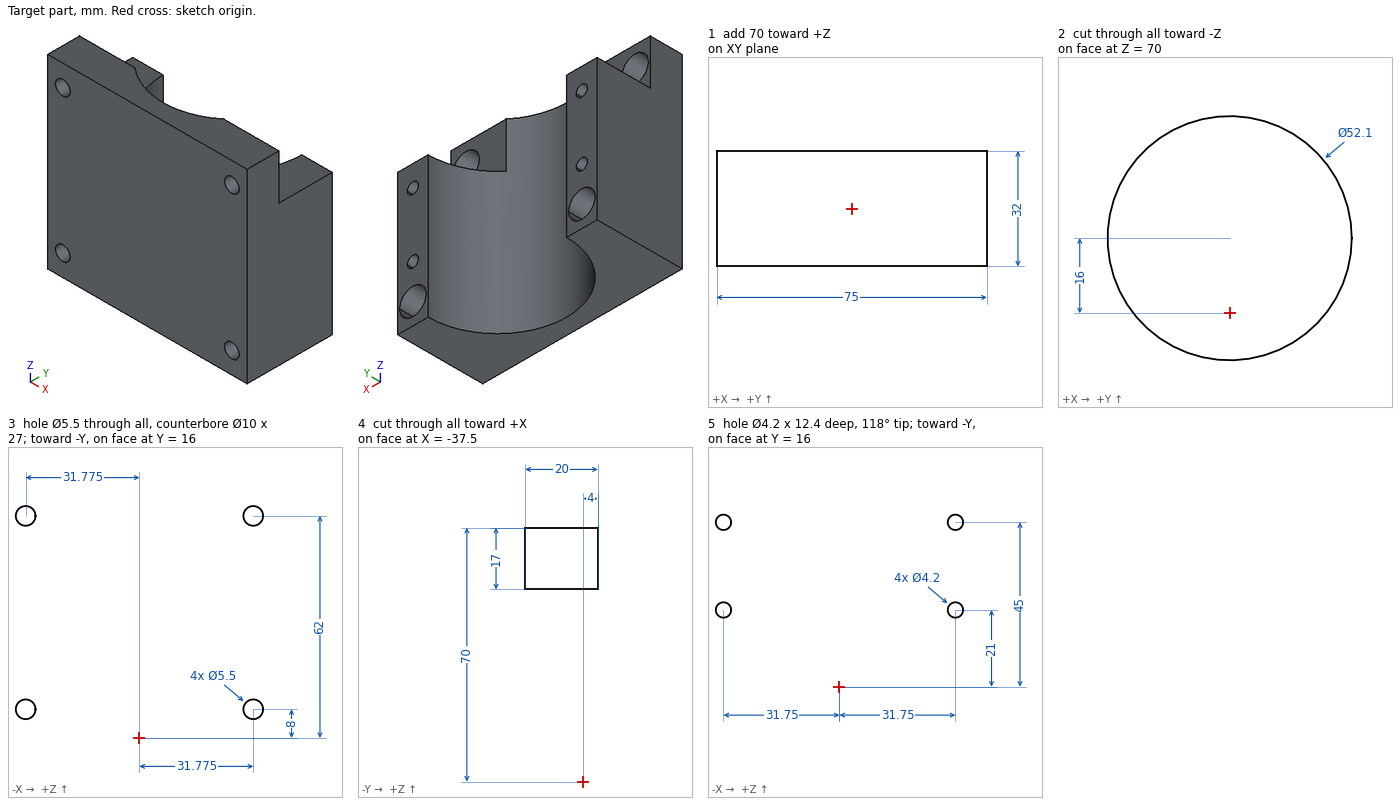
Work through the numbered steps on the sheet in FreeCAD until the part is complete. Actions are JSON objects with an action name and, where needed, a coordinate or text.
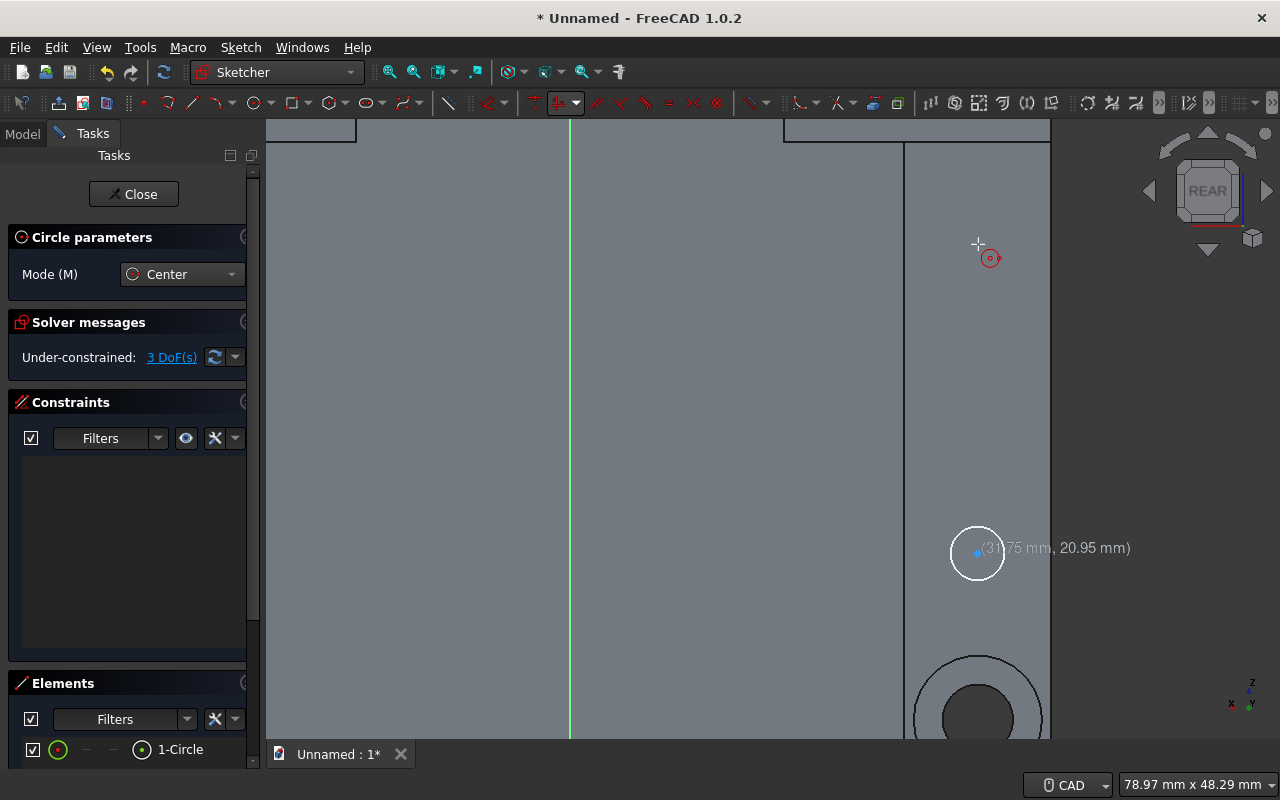
{"action": "left_click", "coordinate": [978, 245]}
{"action": "left_click", "coordinate": [997, 226]}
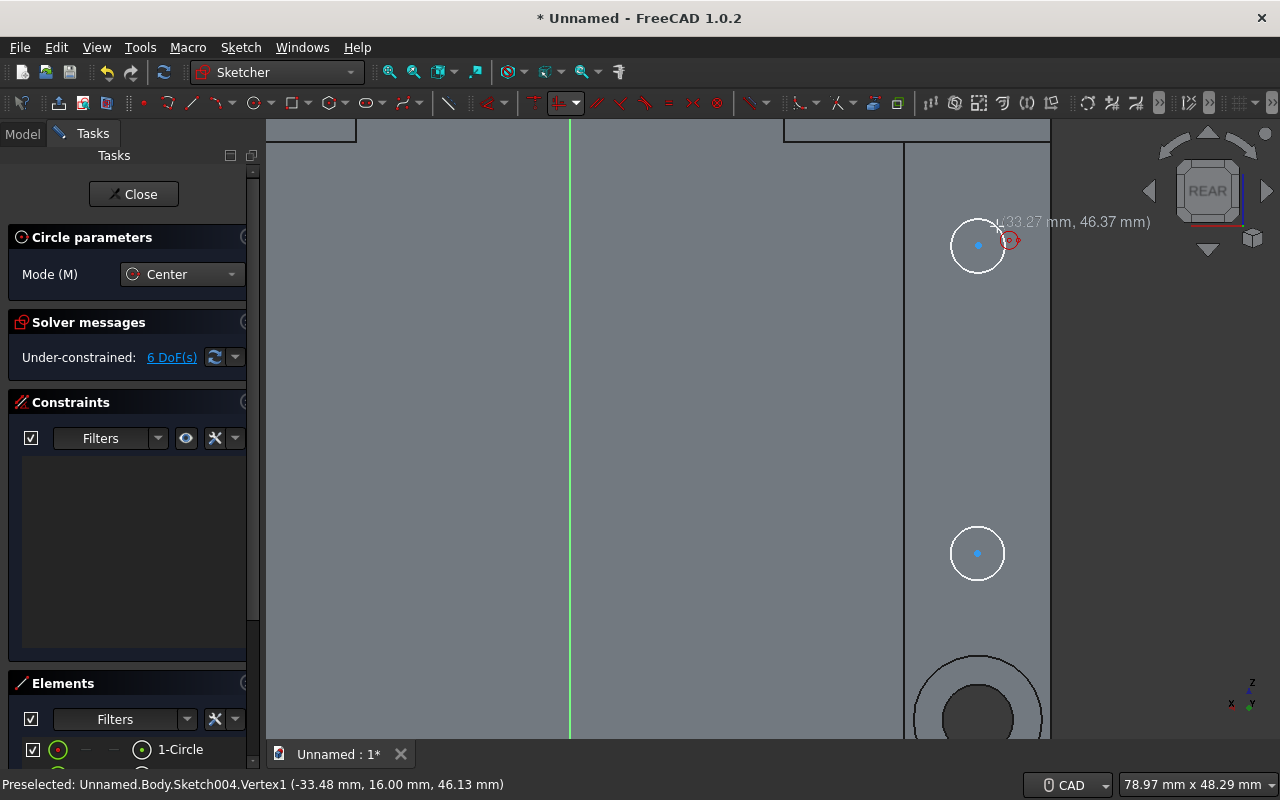
{"action": "scroll", "coordinate": [978, 244], "scroll_direction": "down", "scroll_amount": 2}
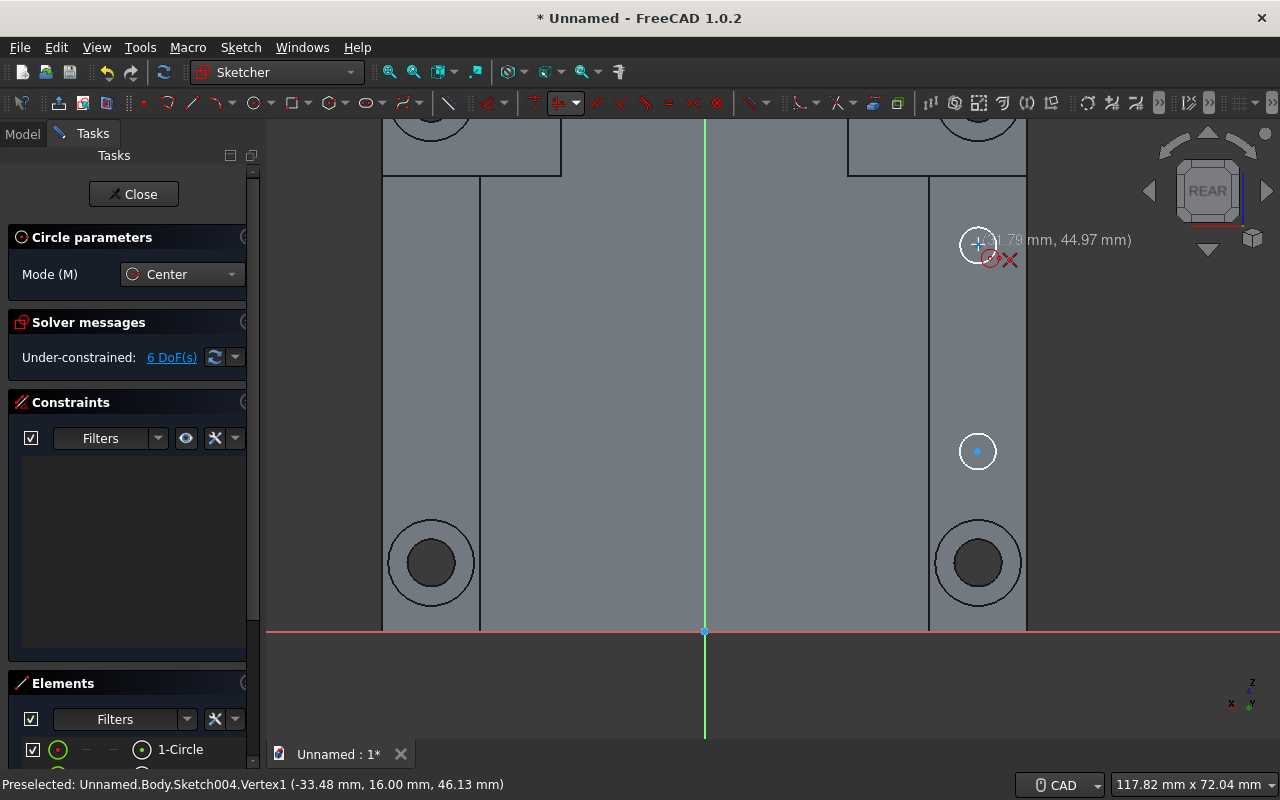
{"action": "scroll", "coordinate": [431, 451], "scroll_direction": "up", "scroll_amount": 2}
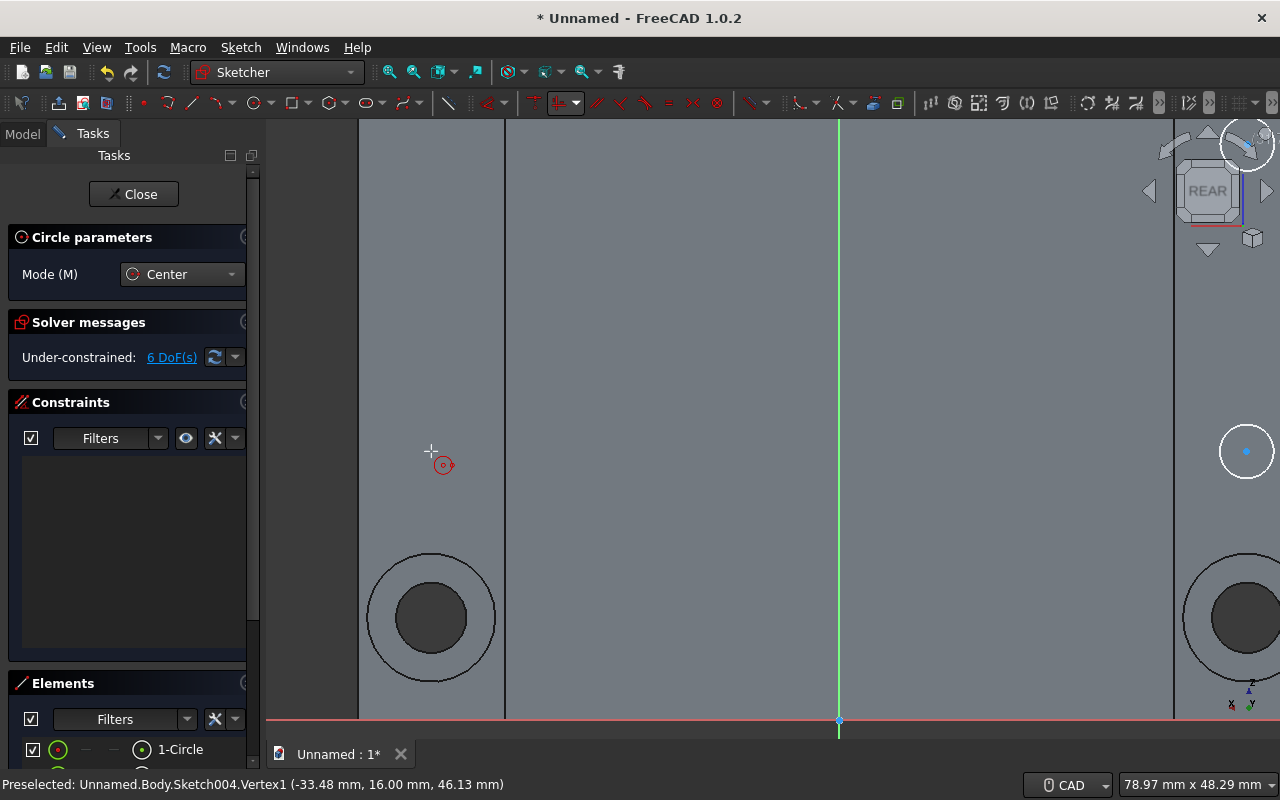
{"action": "left_click", "coordinate": [432, 451]}
{"action": "left_click", "coordinate": [451, 432]}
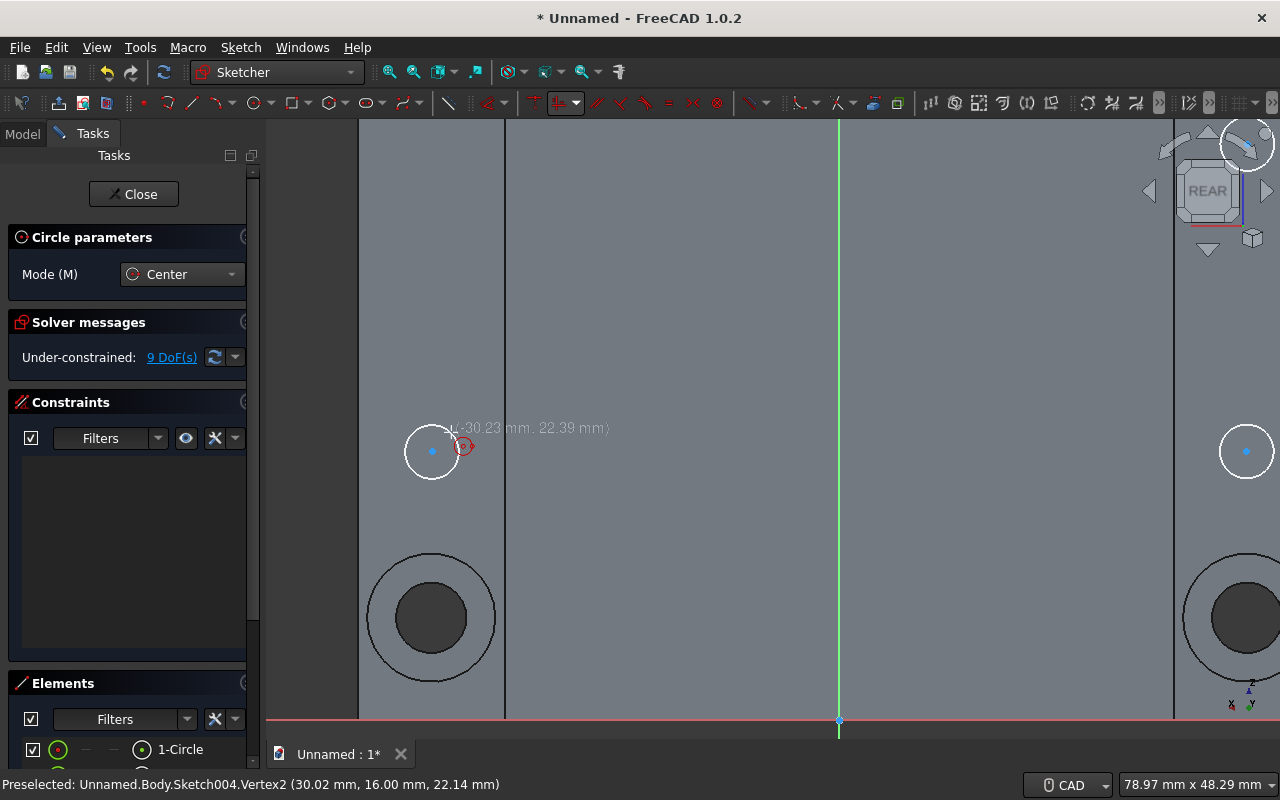
{"action": "scroll", "coordinate": [431, 451], "scroll_direction": "down", "scroll_amount": 2}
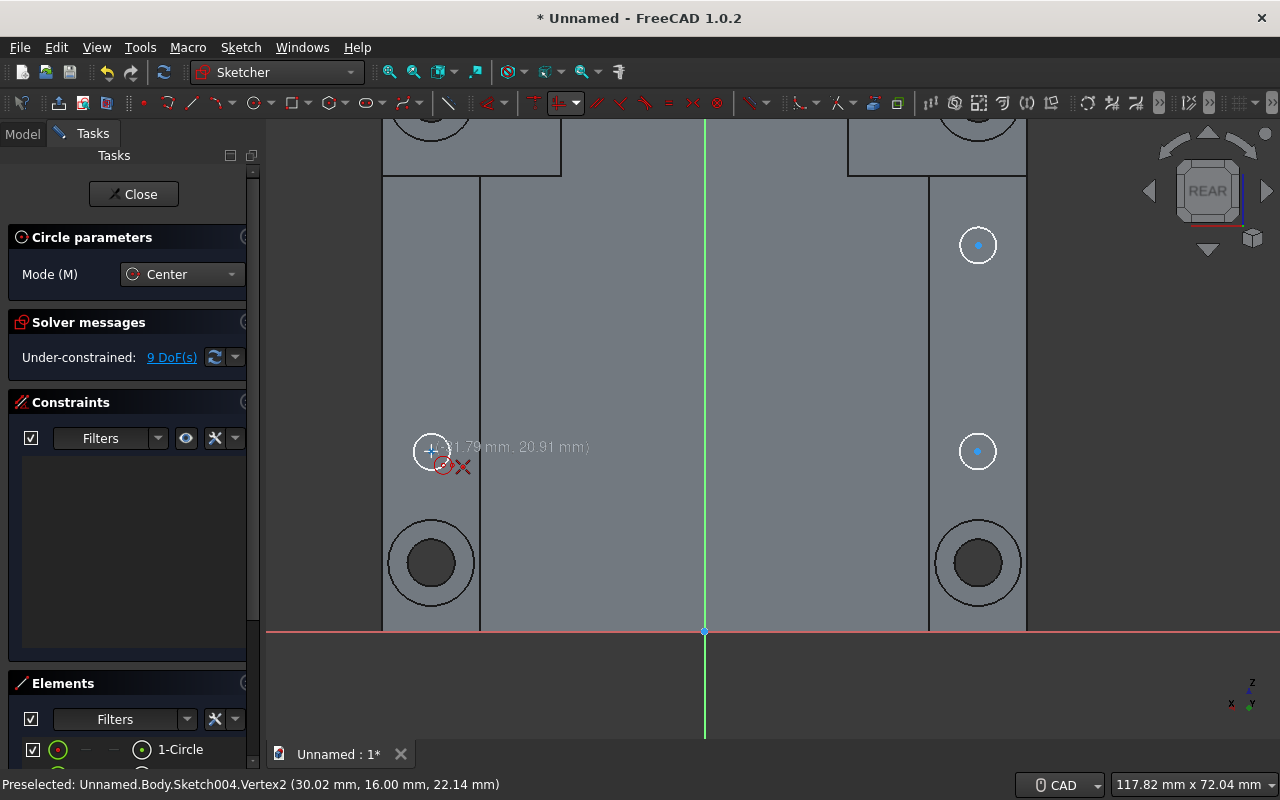
{"action": "scroll", "coordinate": [431, 244], "scroll_direction": "up", "scroll_amount": 2}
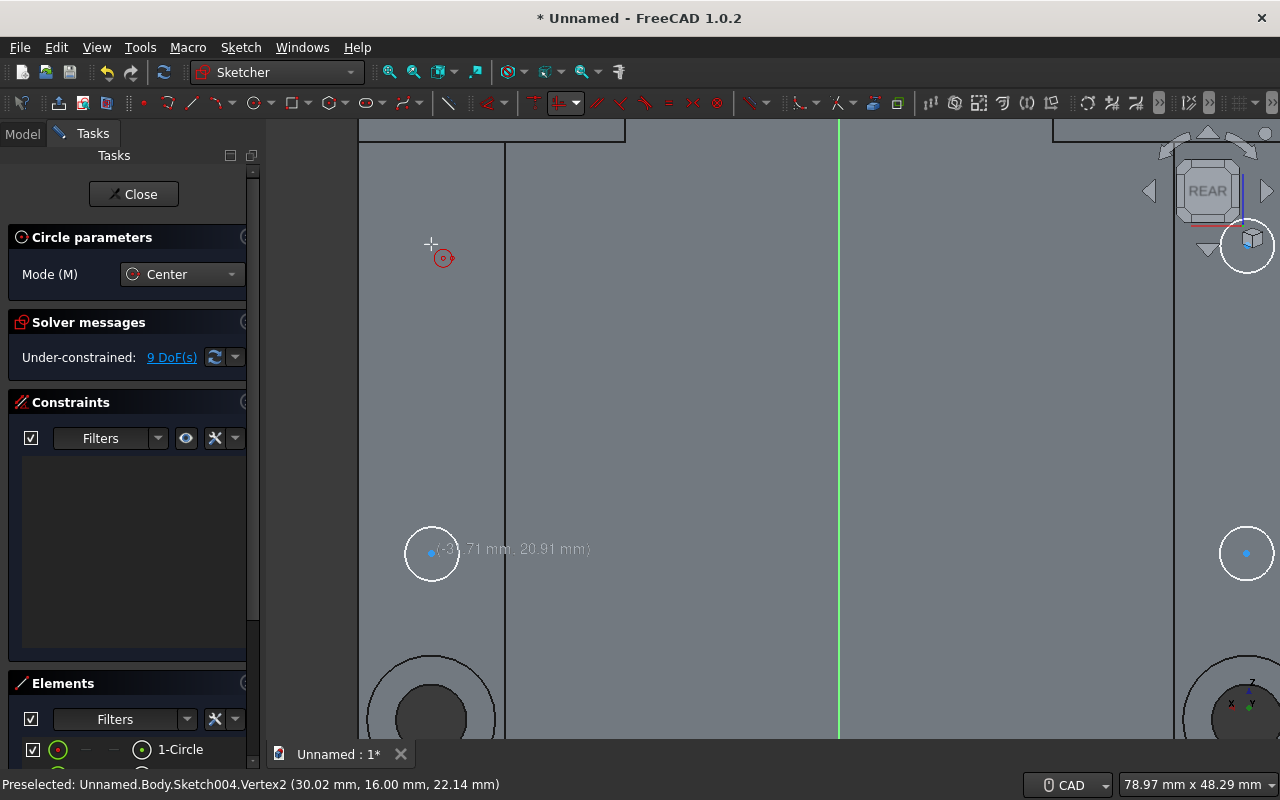
{"action": "left_click", "coordinate": [432, 245]}
{"action": "left_click", "coordinate": [451, 226]}
{"action": "key", "text": "Escape"}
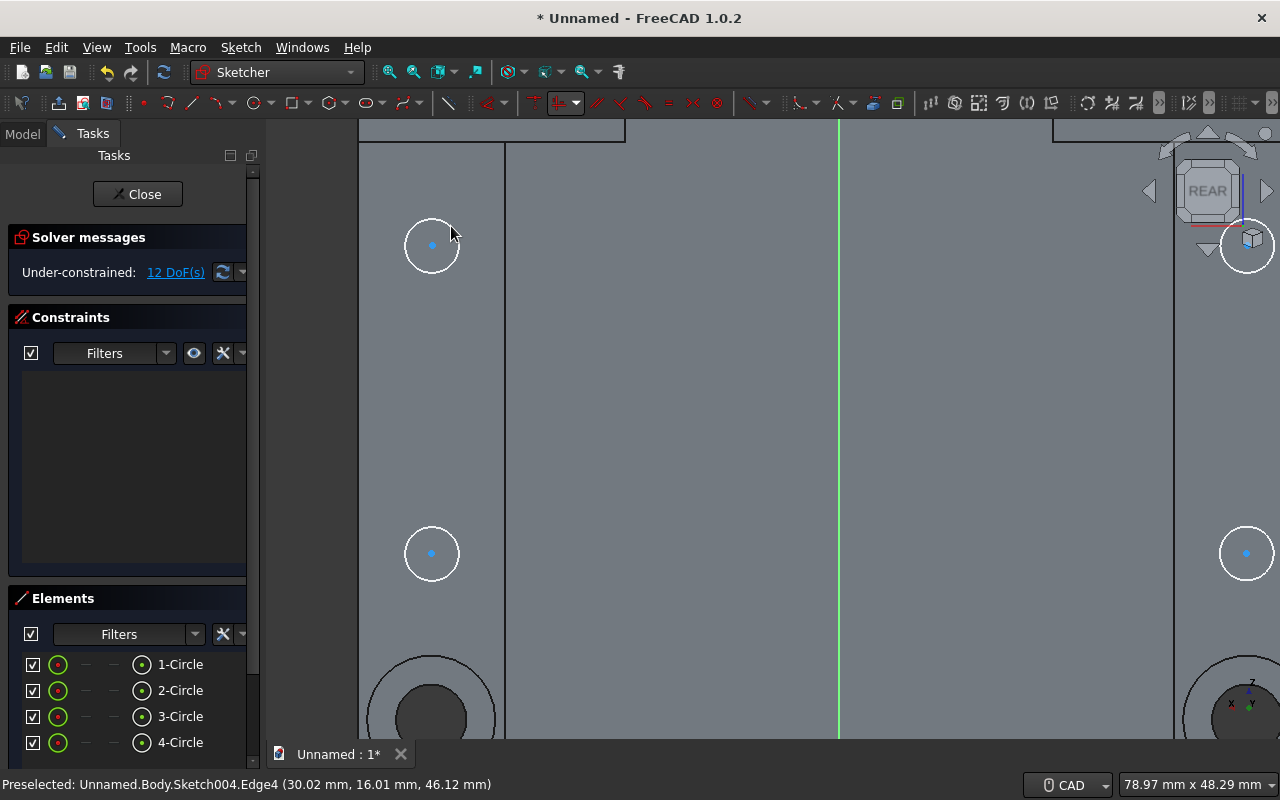
{"action": "scroll", "coordinate": [431, 244], "scroll_direction": "down", "scroll_amount": 2}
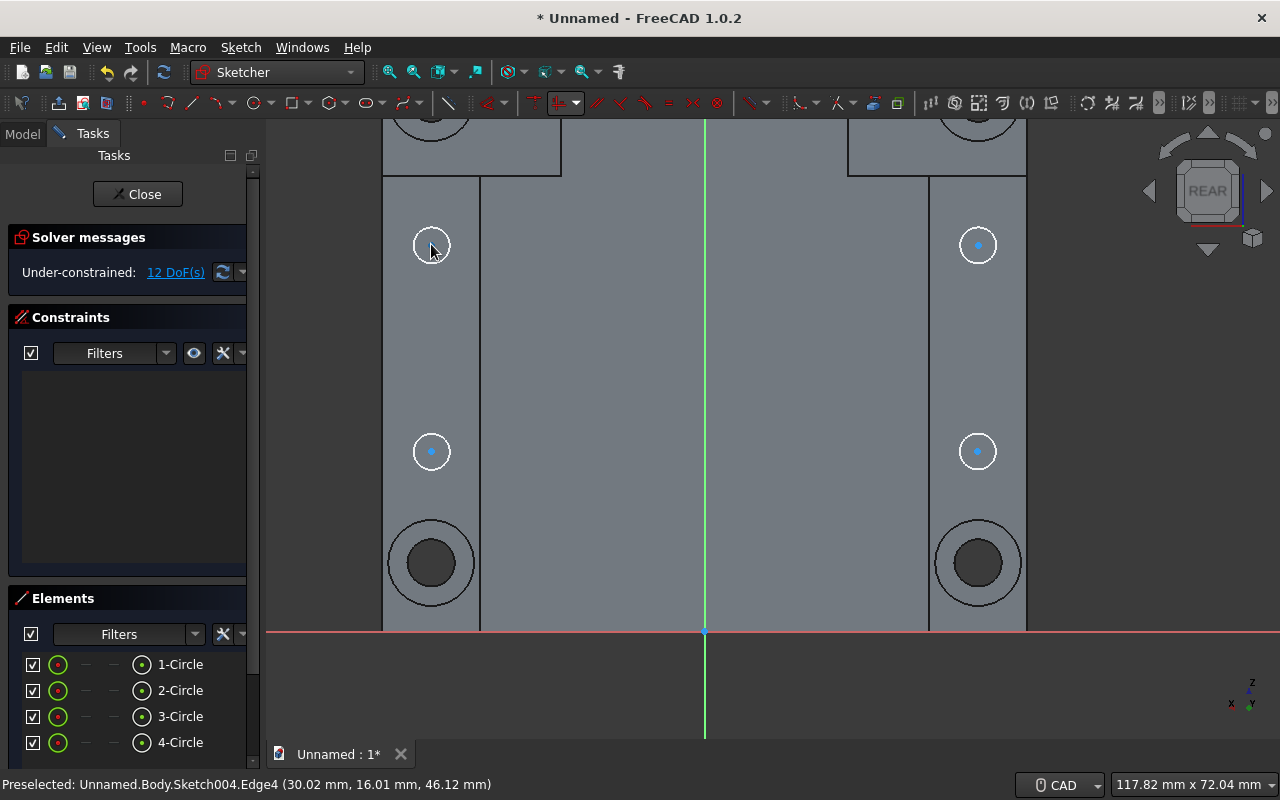
{"action": "left_click", "coordinate": [991, 439]}